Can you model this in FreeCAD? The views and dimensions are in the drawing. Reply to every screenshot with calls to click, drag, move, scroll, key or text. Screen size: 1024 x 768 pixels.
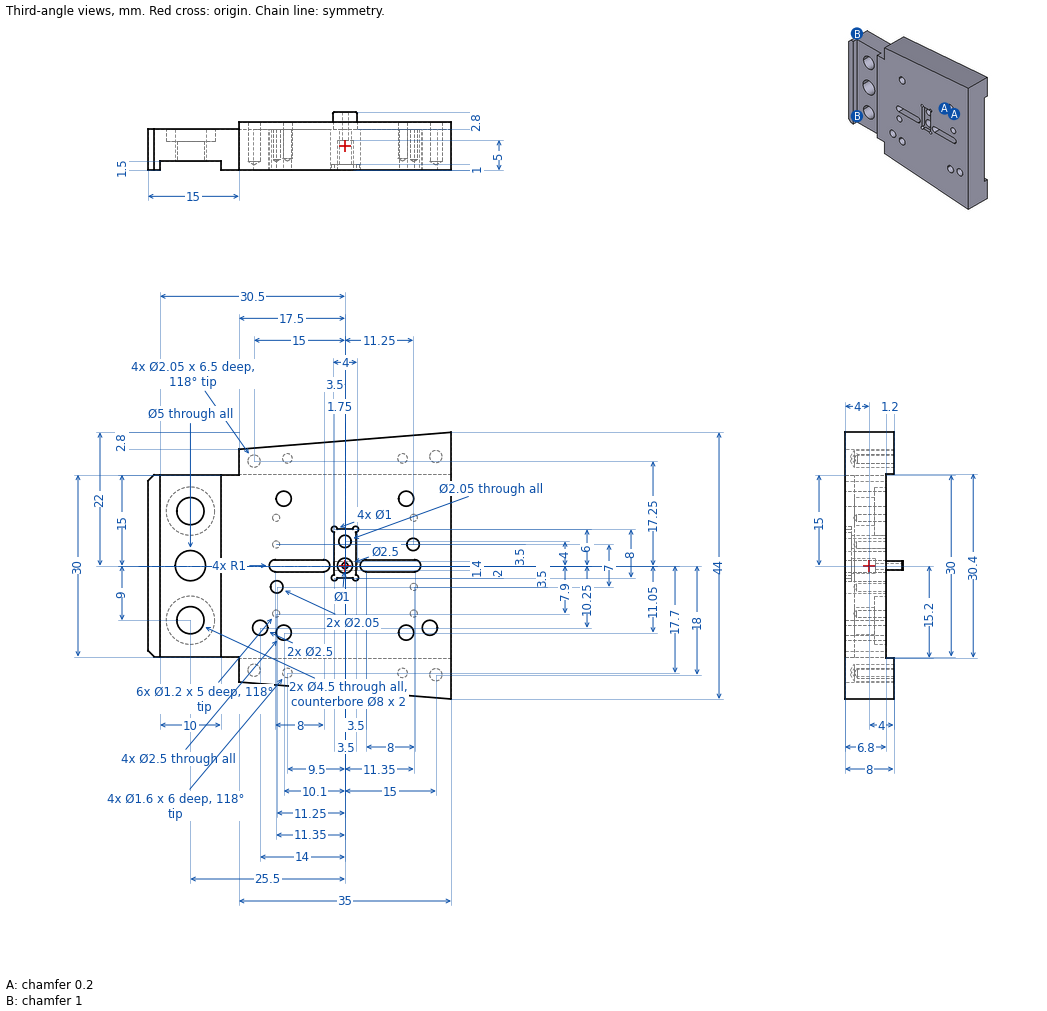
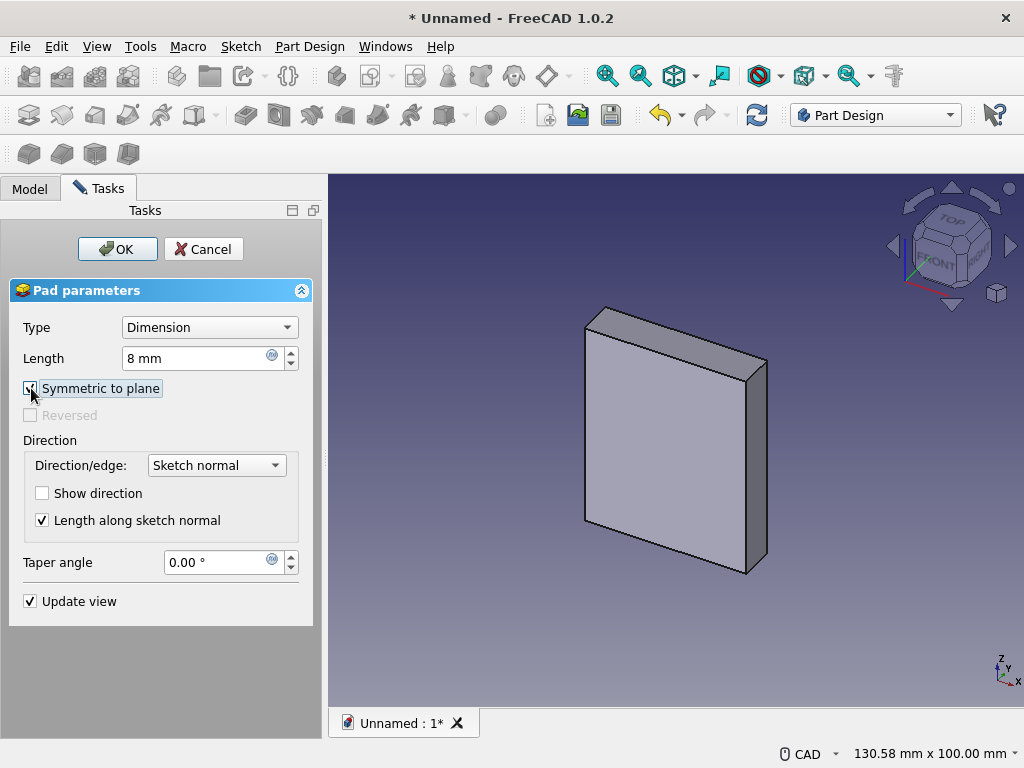
click(118, 249)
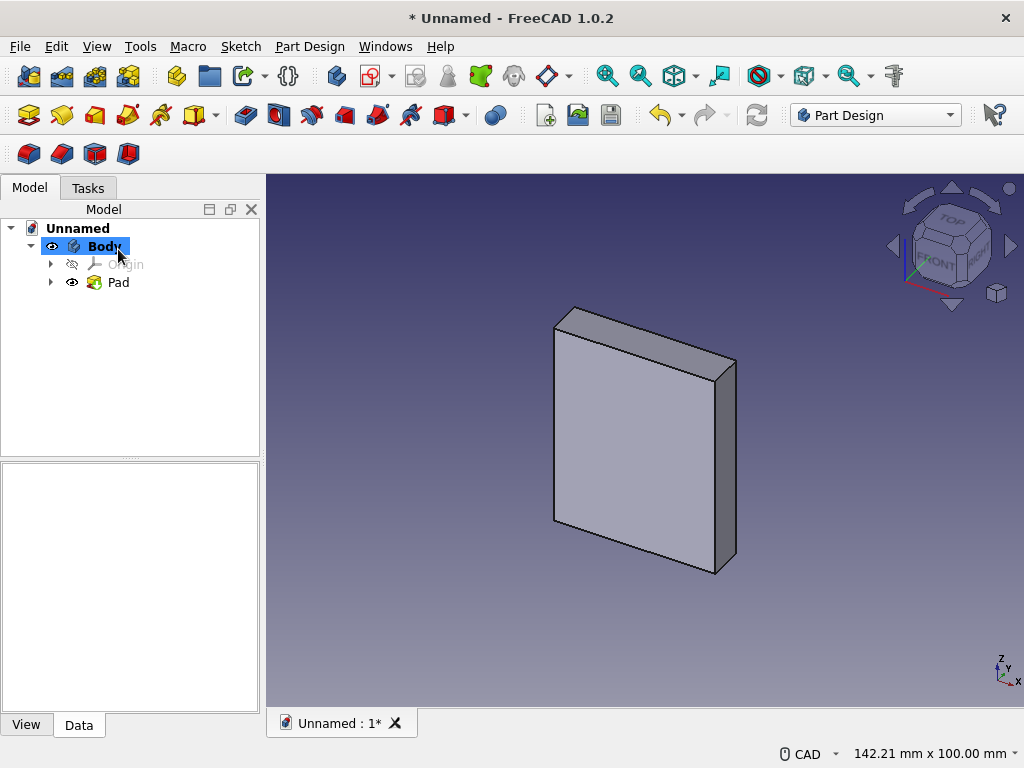
key(4)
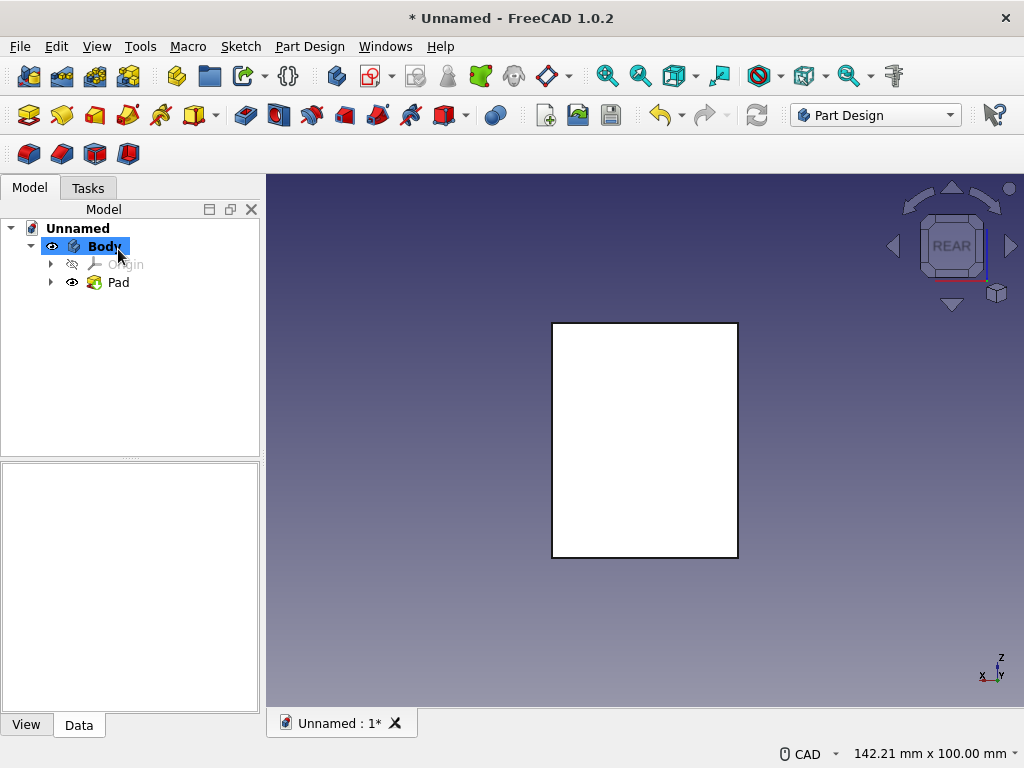
click(608, 76)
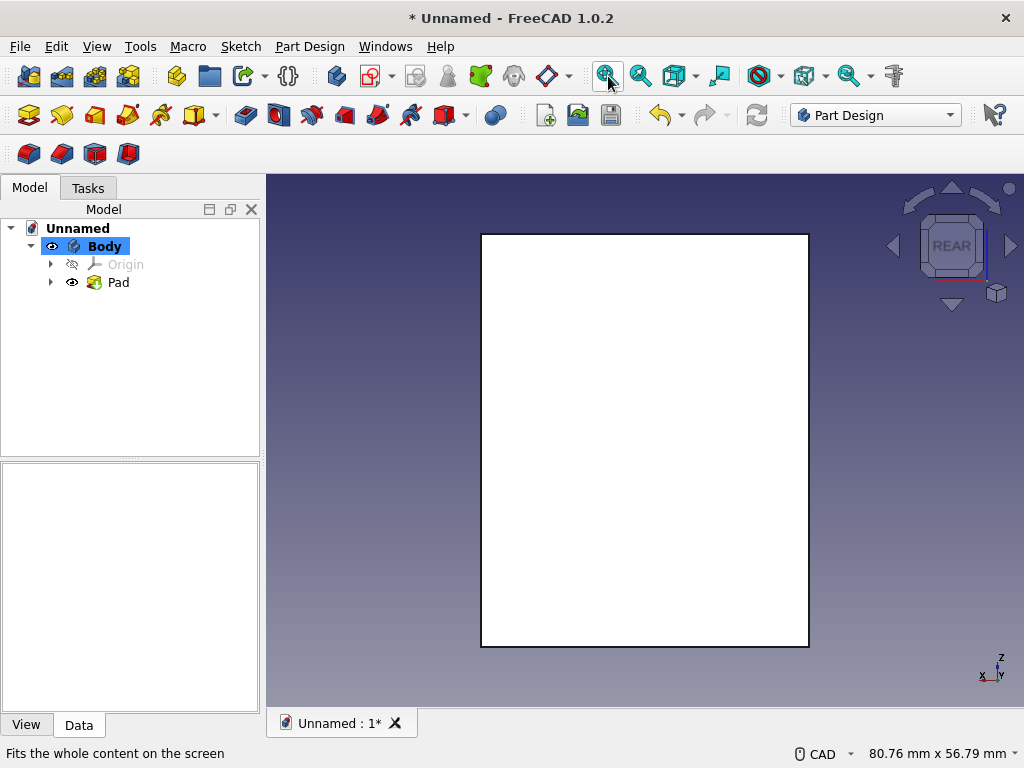
click(645, 440)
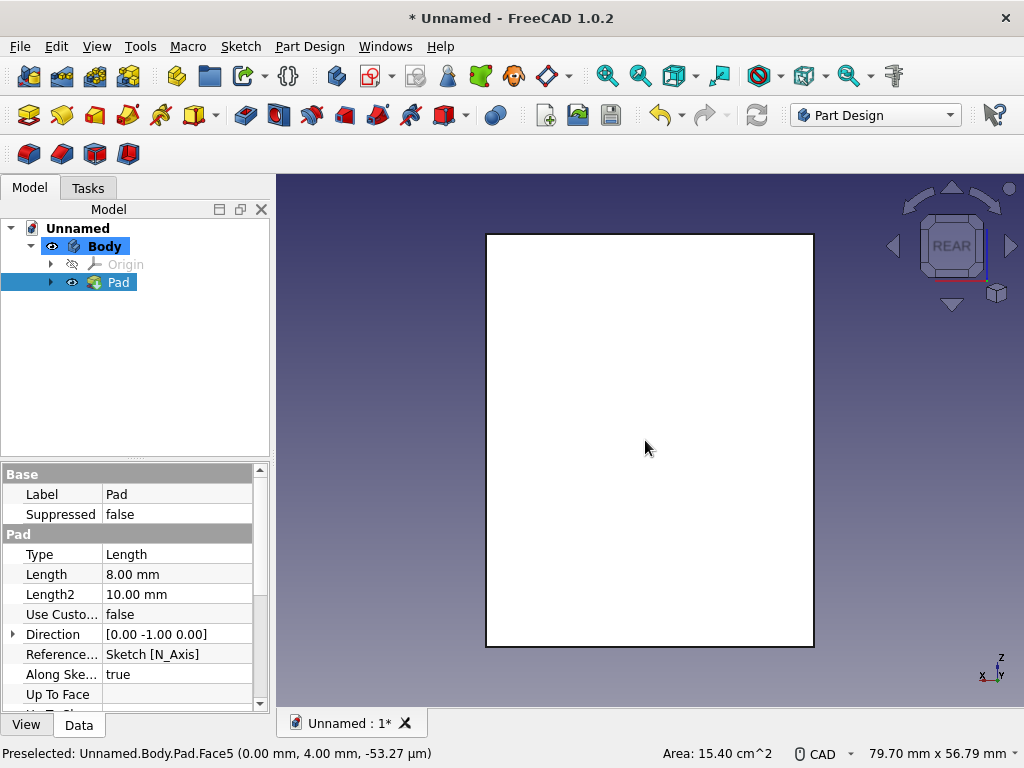
click(370, 76)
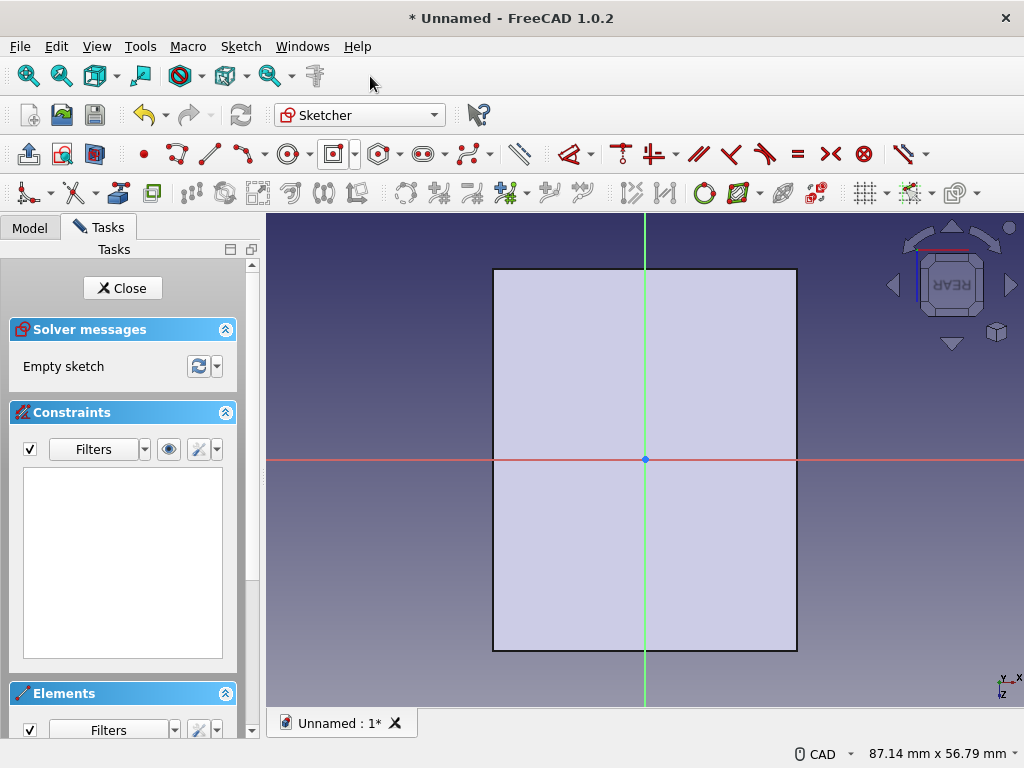
scroll(728, 460, up, 3)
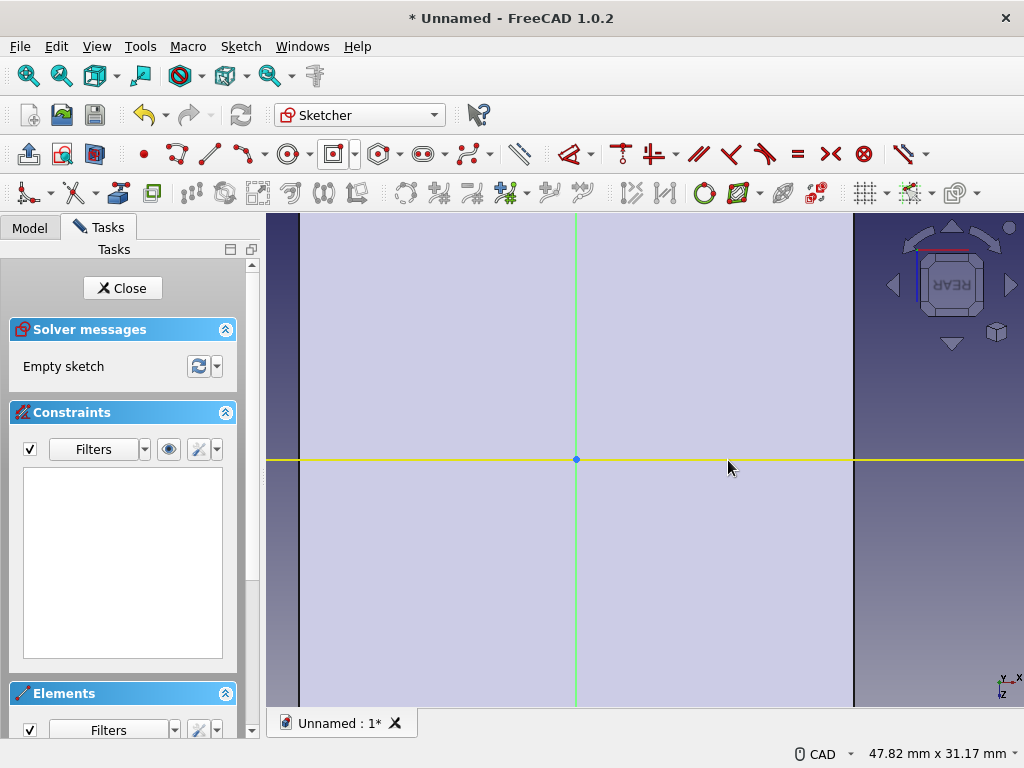
click(422, 154)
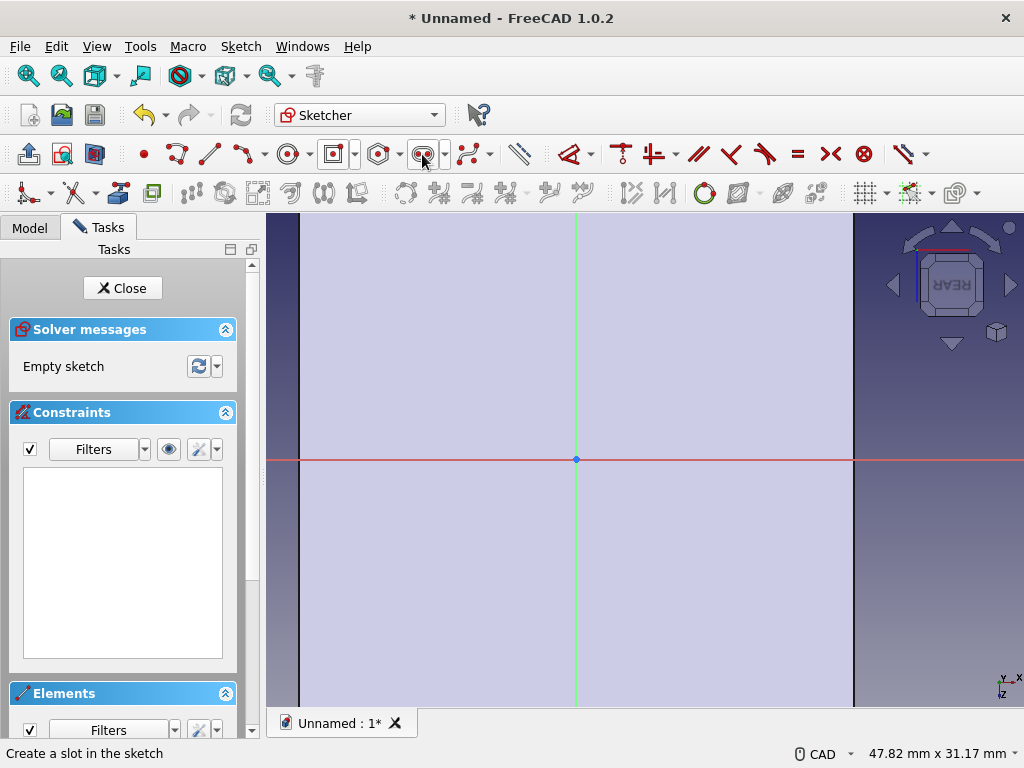
scroll(394, 460, up, 2)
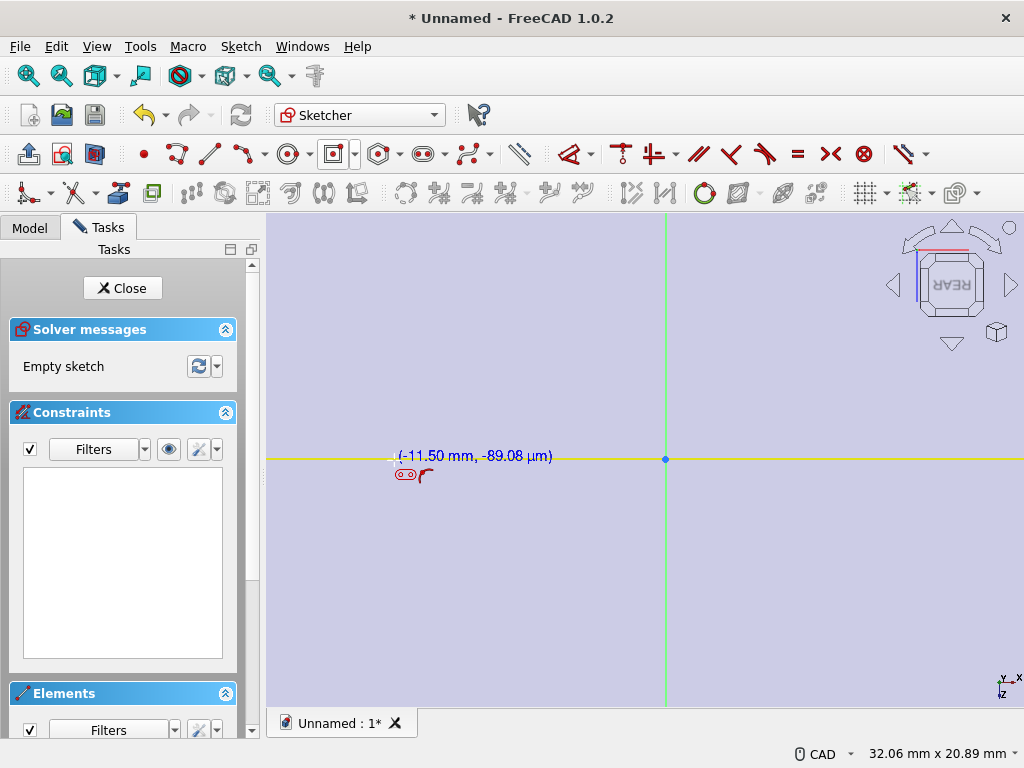
click(394, 459)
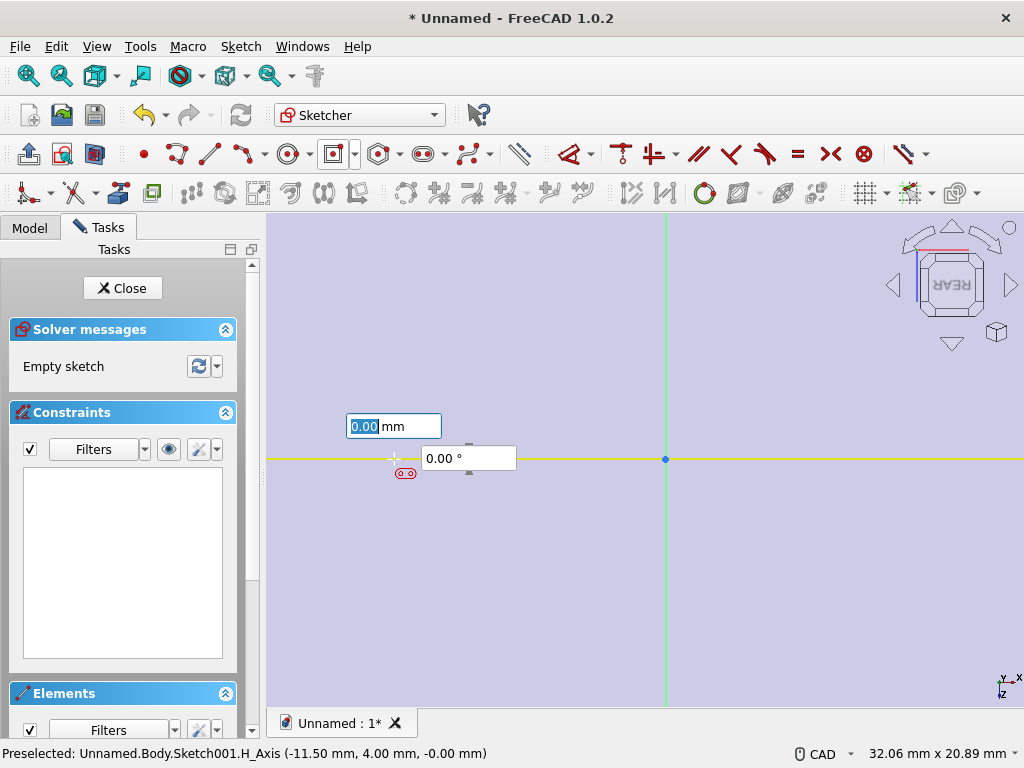
click(583, 450)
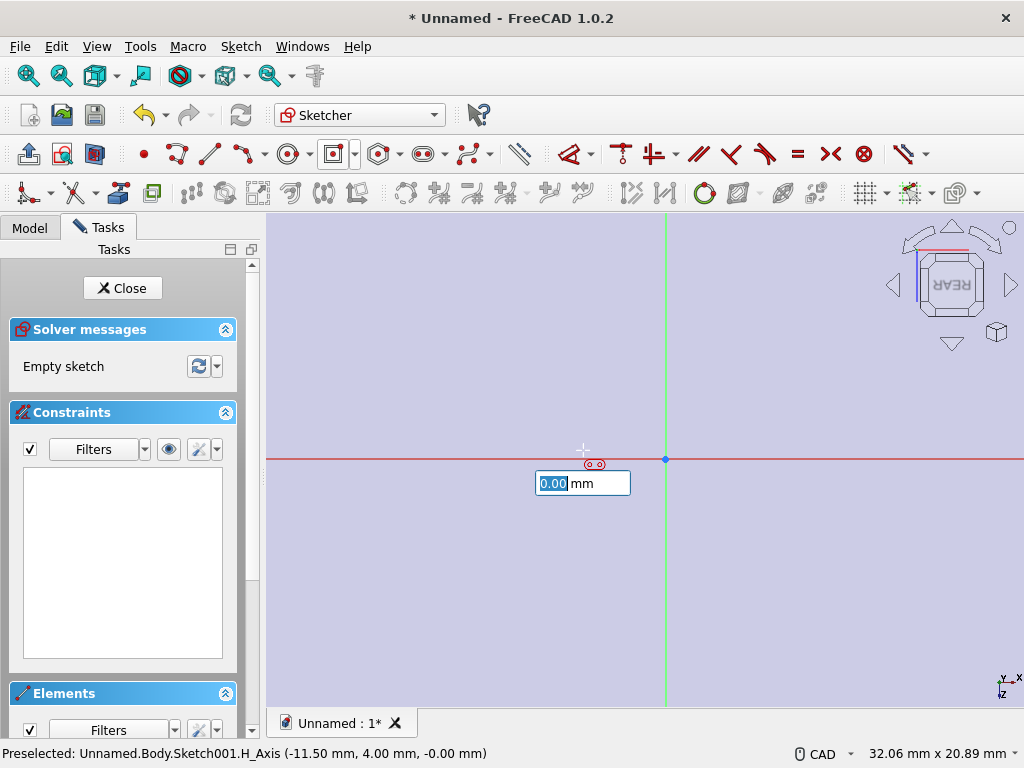
click(488, 435)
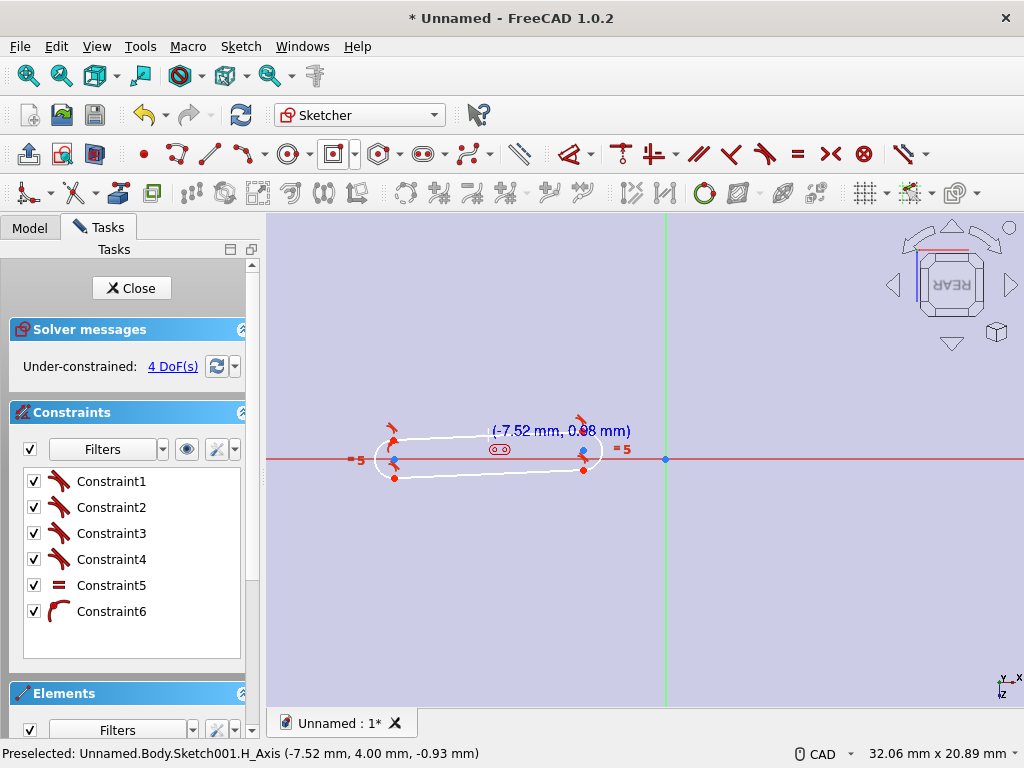
click(749, 459)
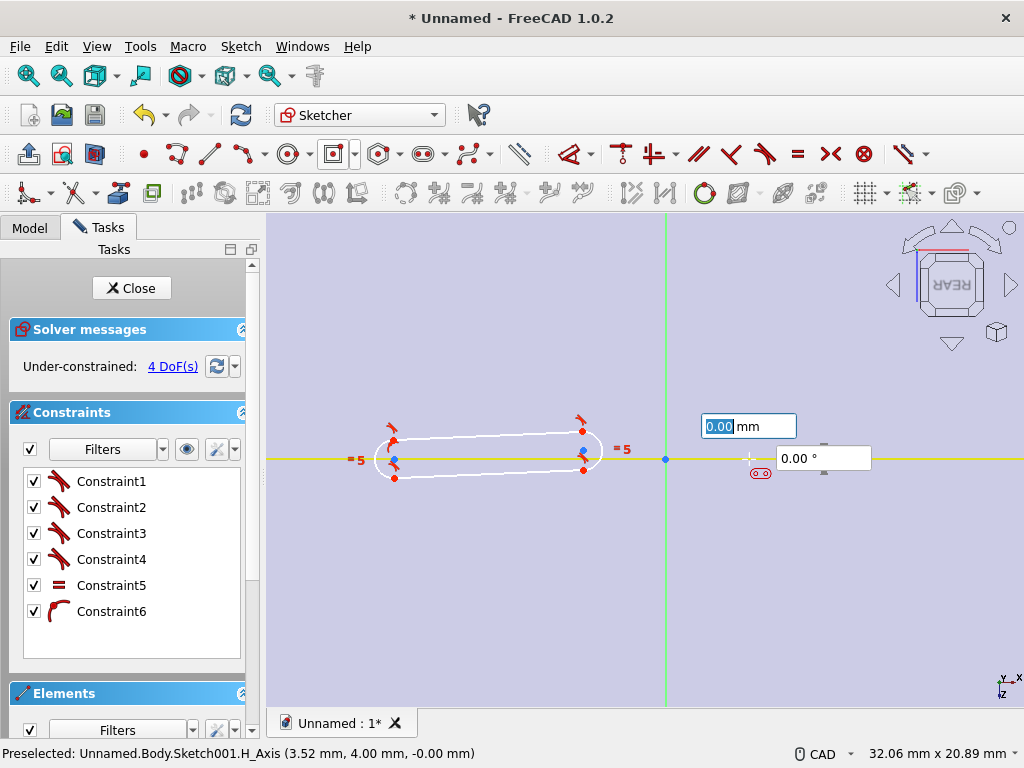
scroll(395, 462, down, 2)